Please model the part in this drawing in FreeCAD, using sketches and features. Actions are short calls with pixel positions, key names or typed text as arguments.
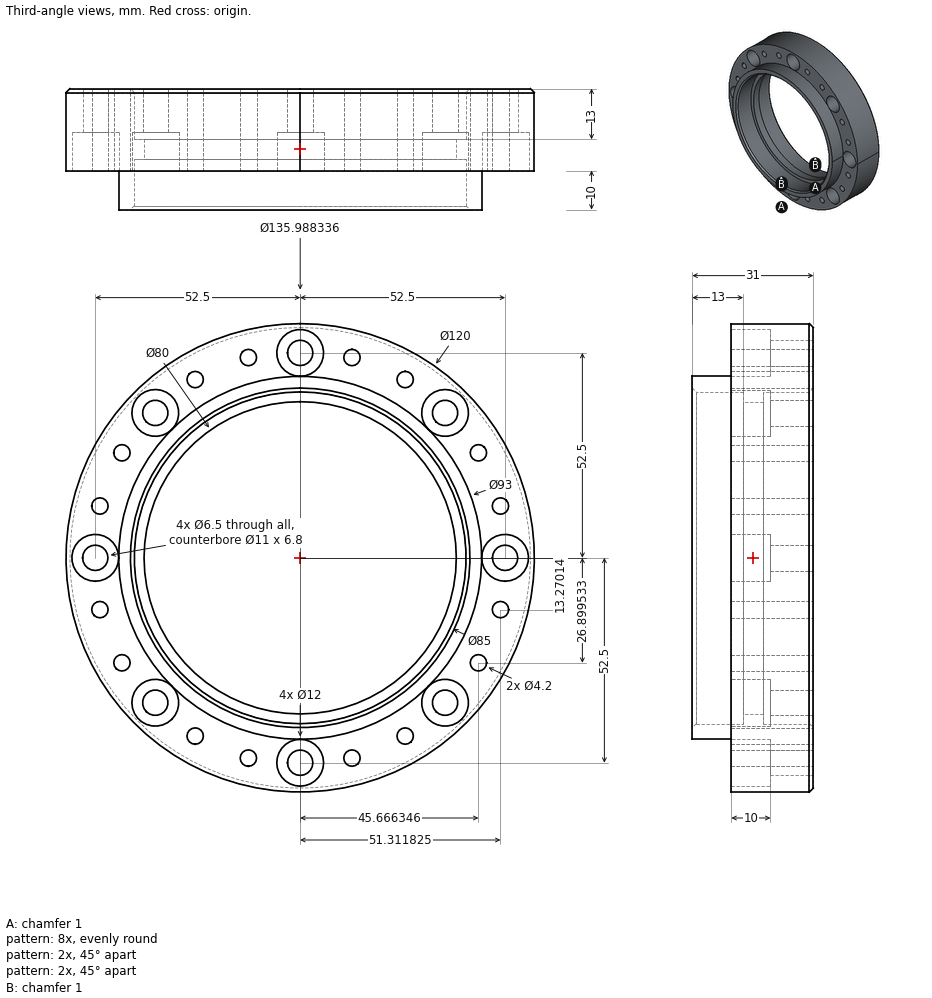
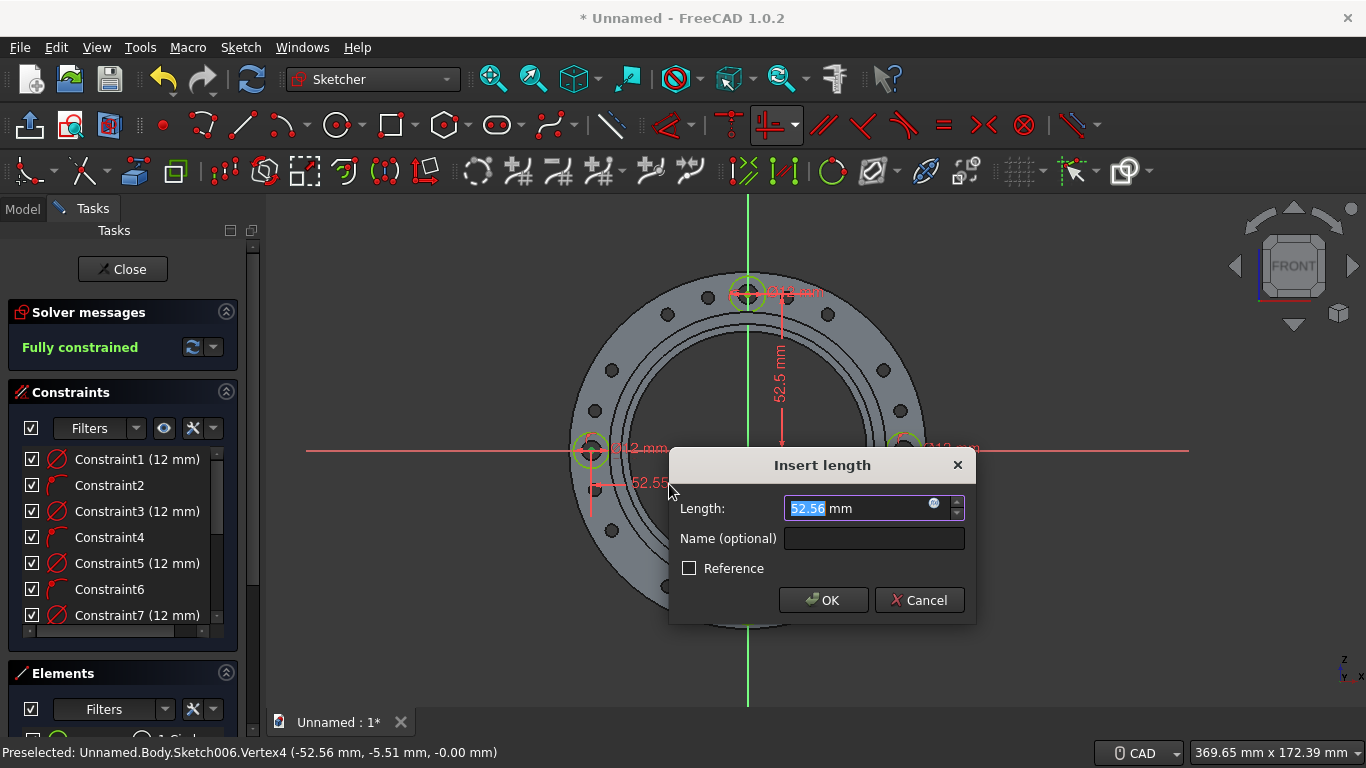
text(52.5)
key(Return)
key(Escape)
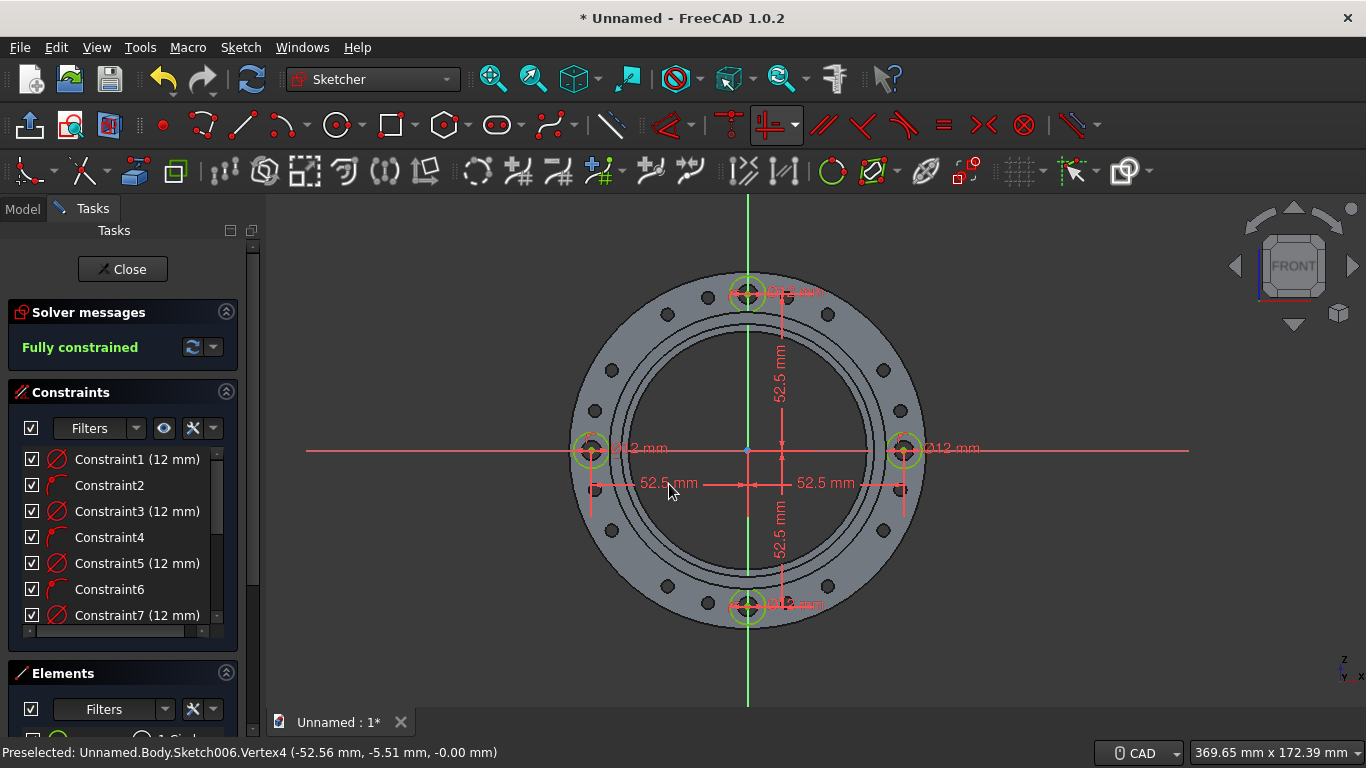
click(123, 269)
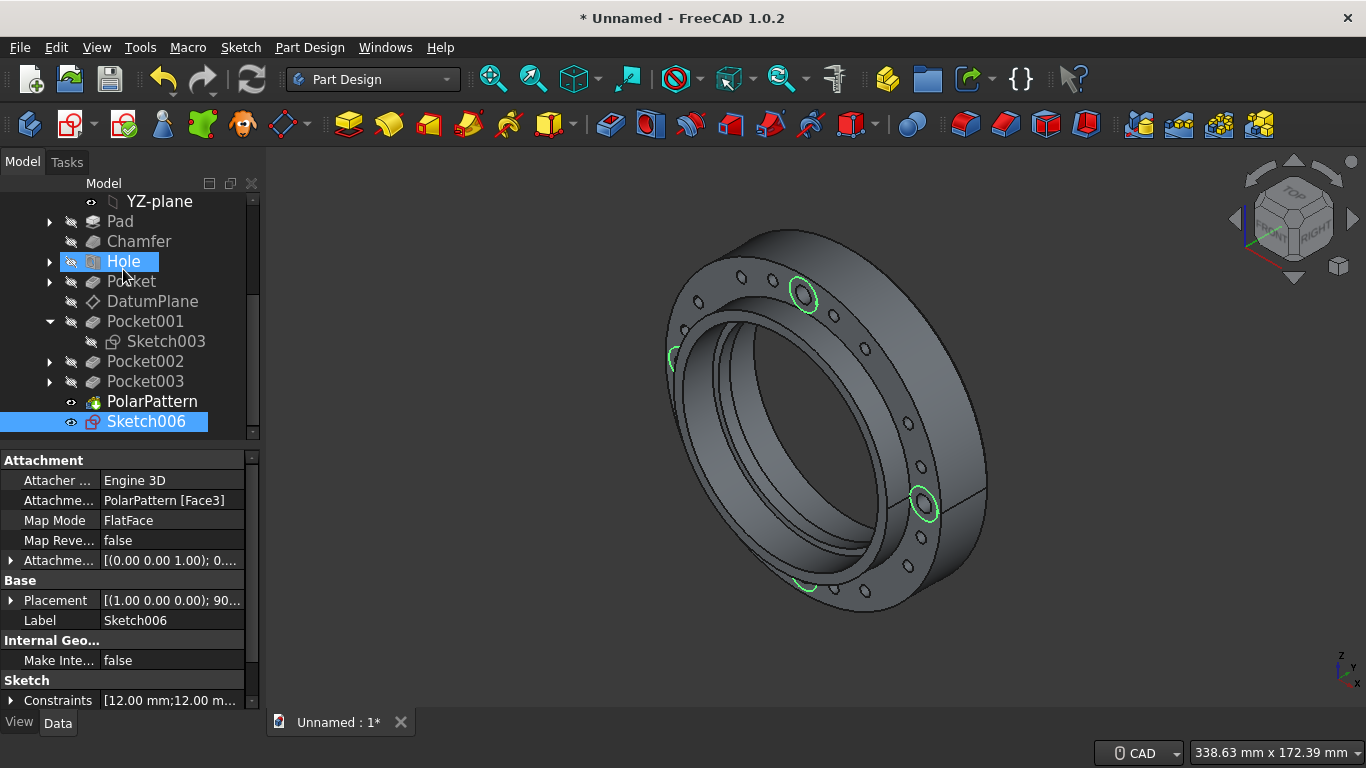
click(612, 124)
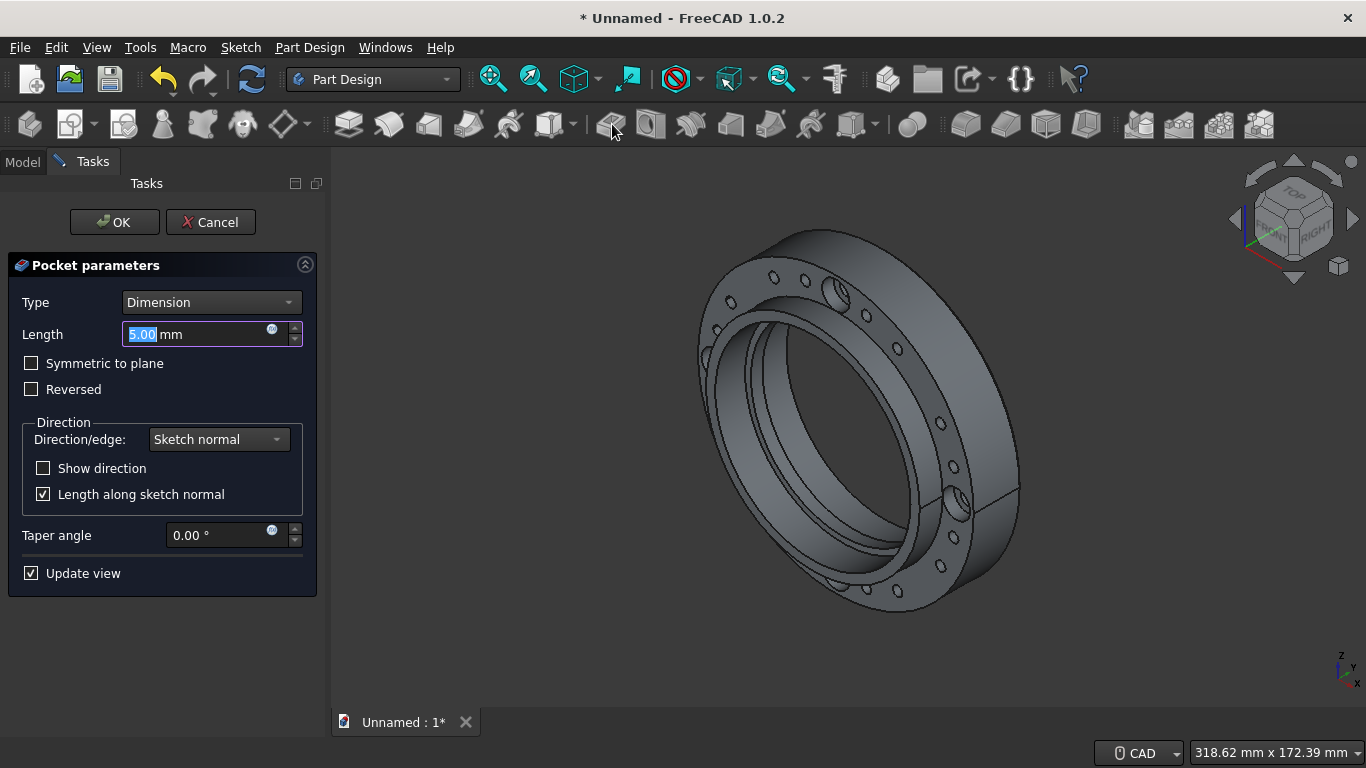
text(10)
key(Tab)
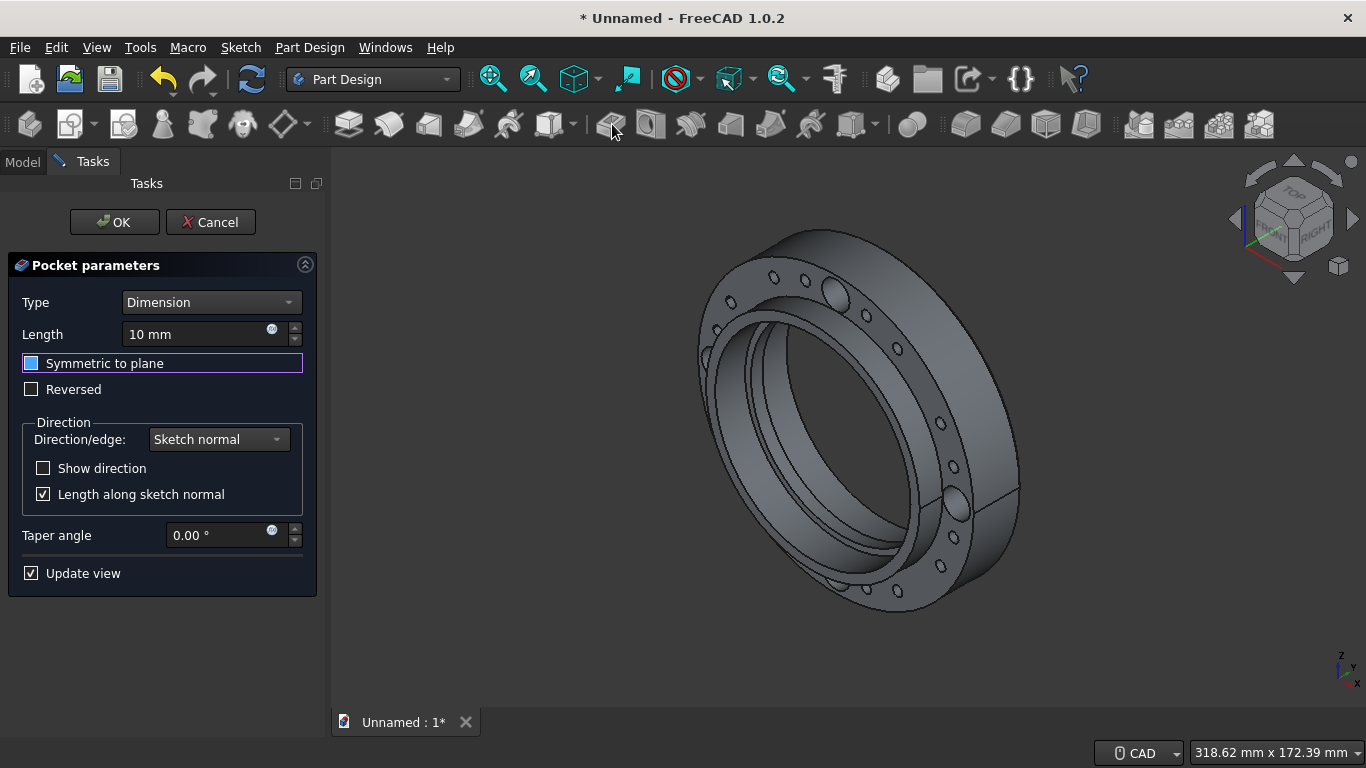
click(115, 222)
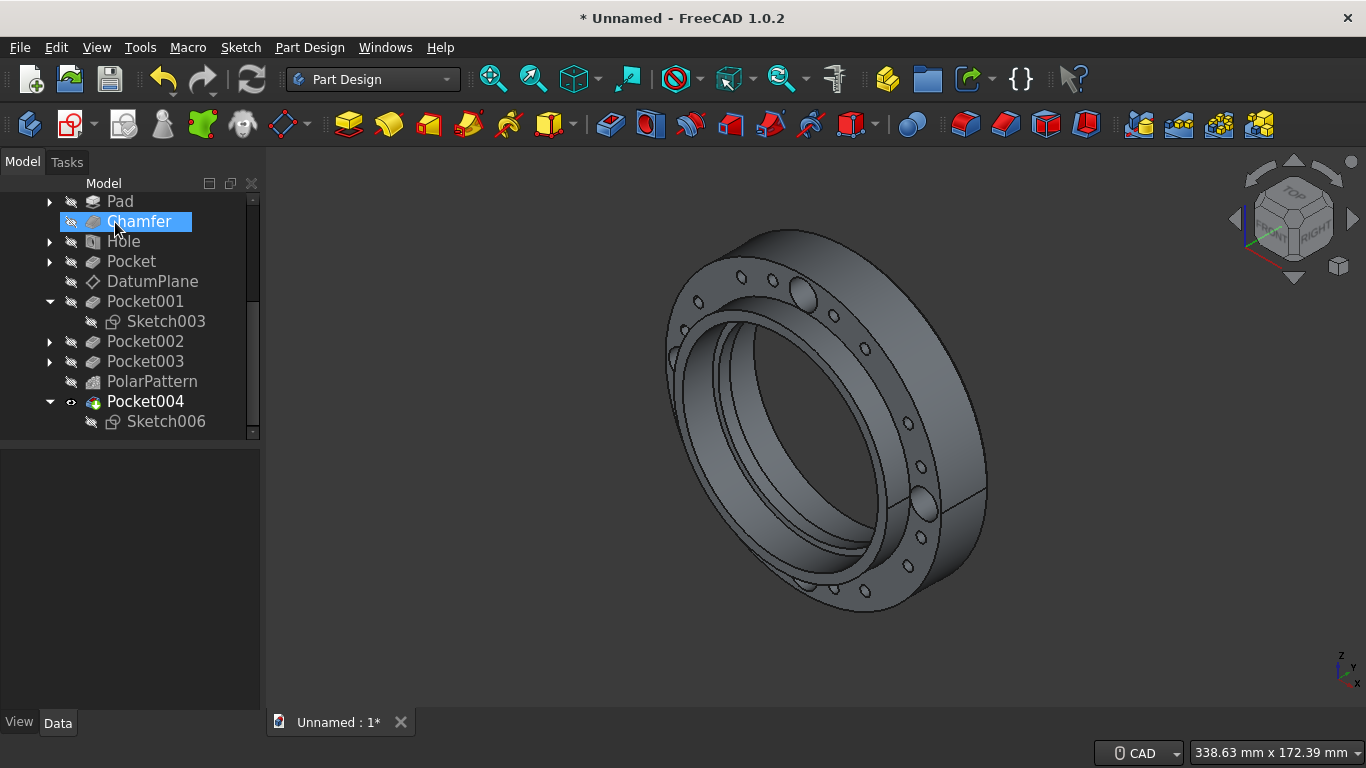
click(116, 242)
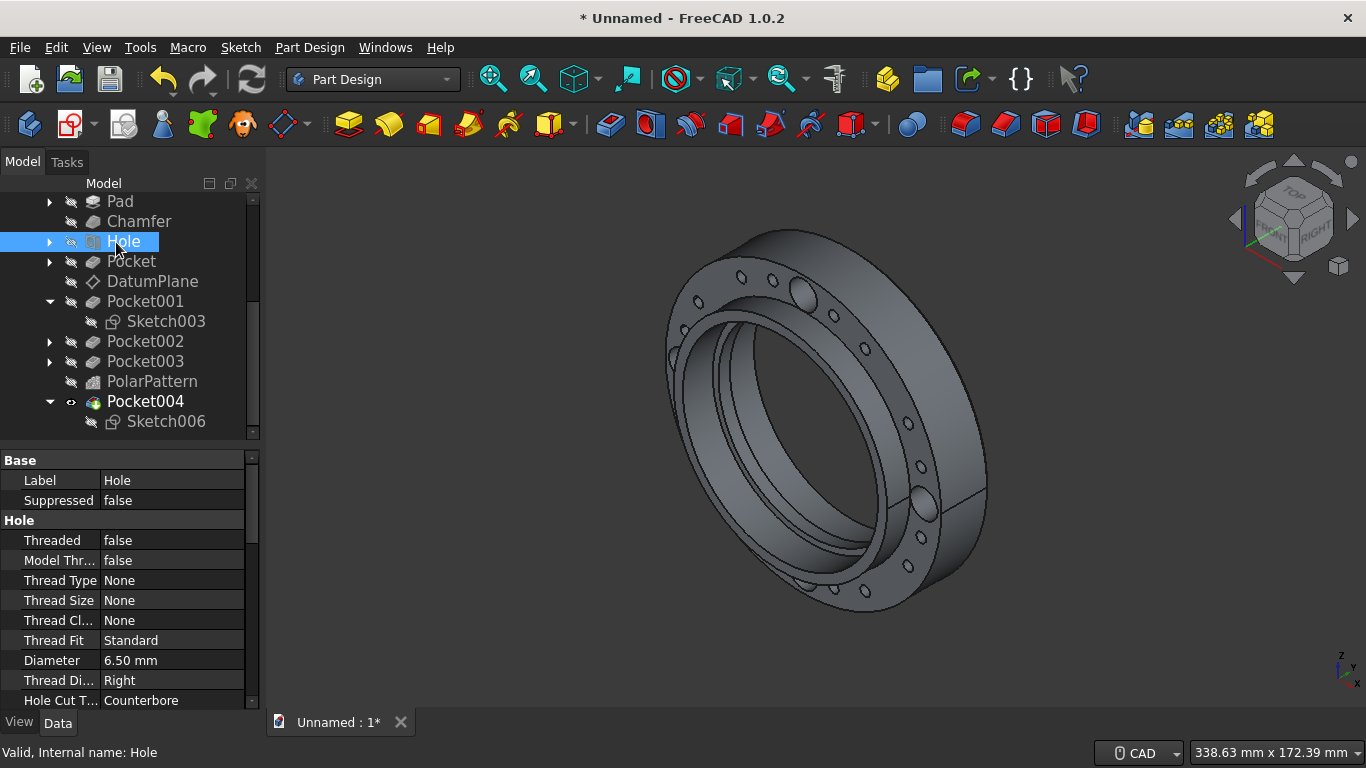
click(1220, 124)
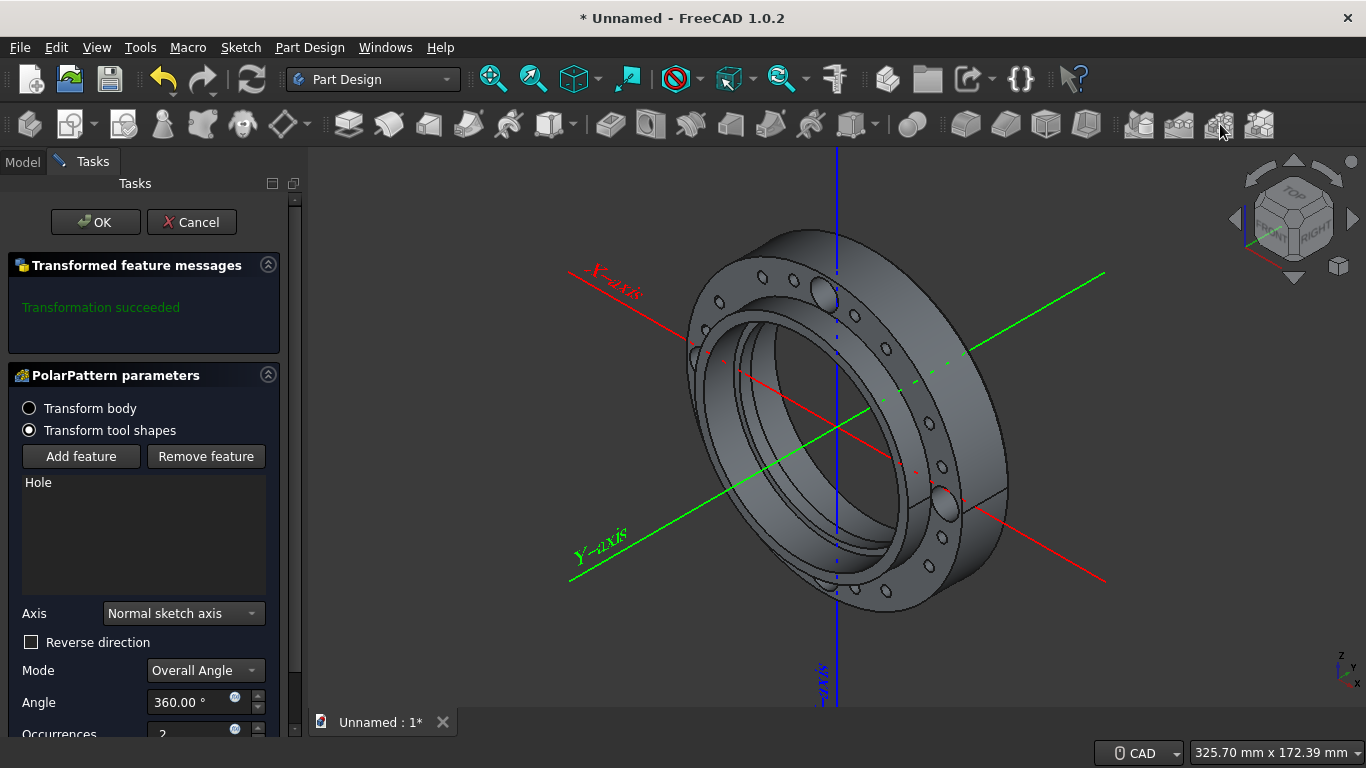
click(184, 614)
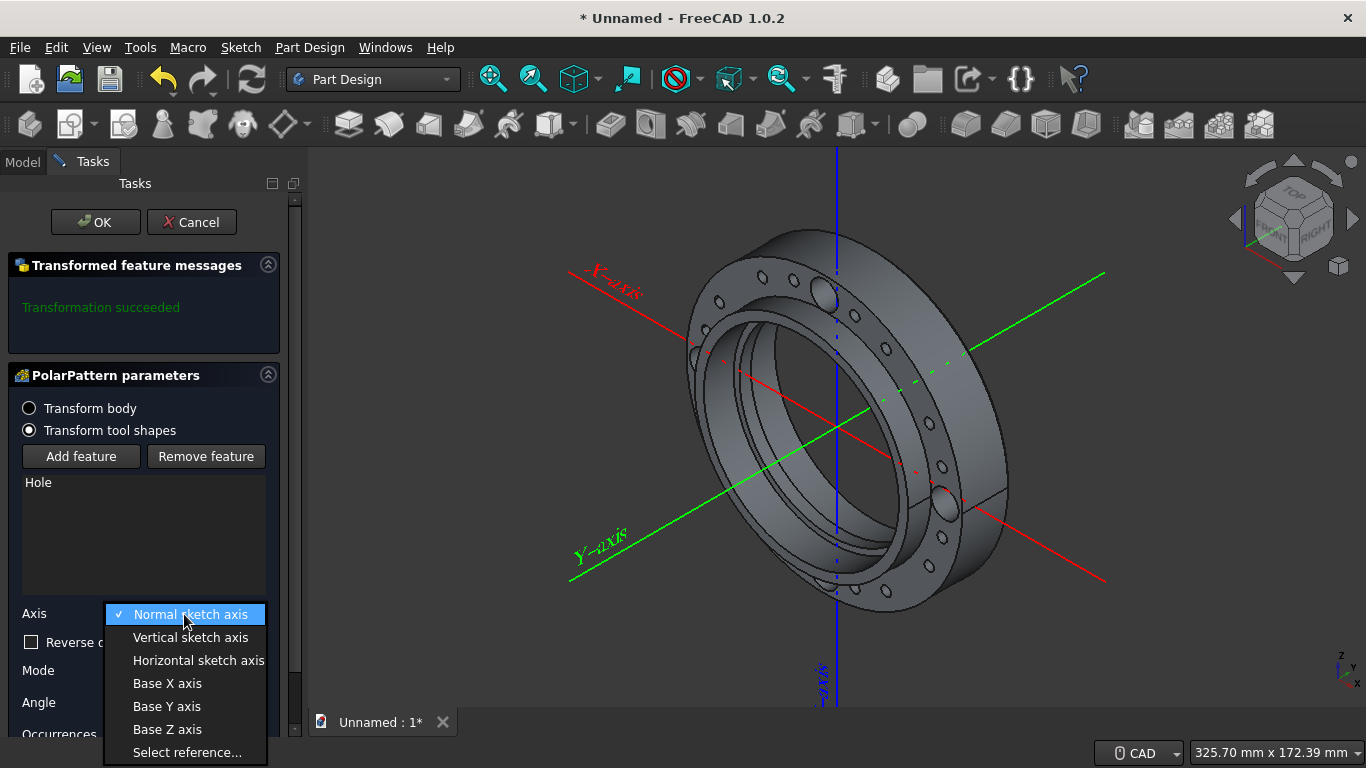
click(184, 706)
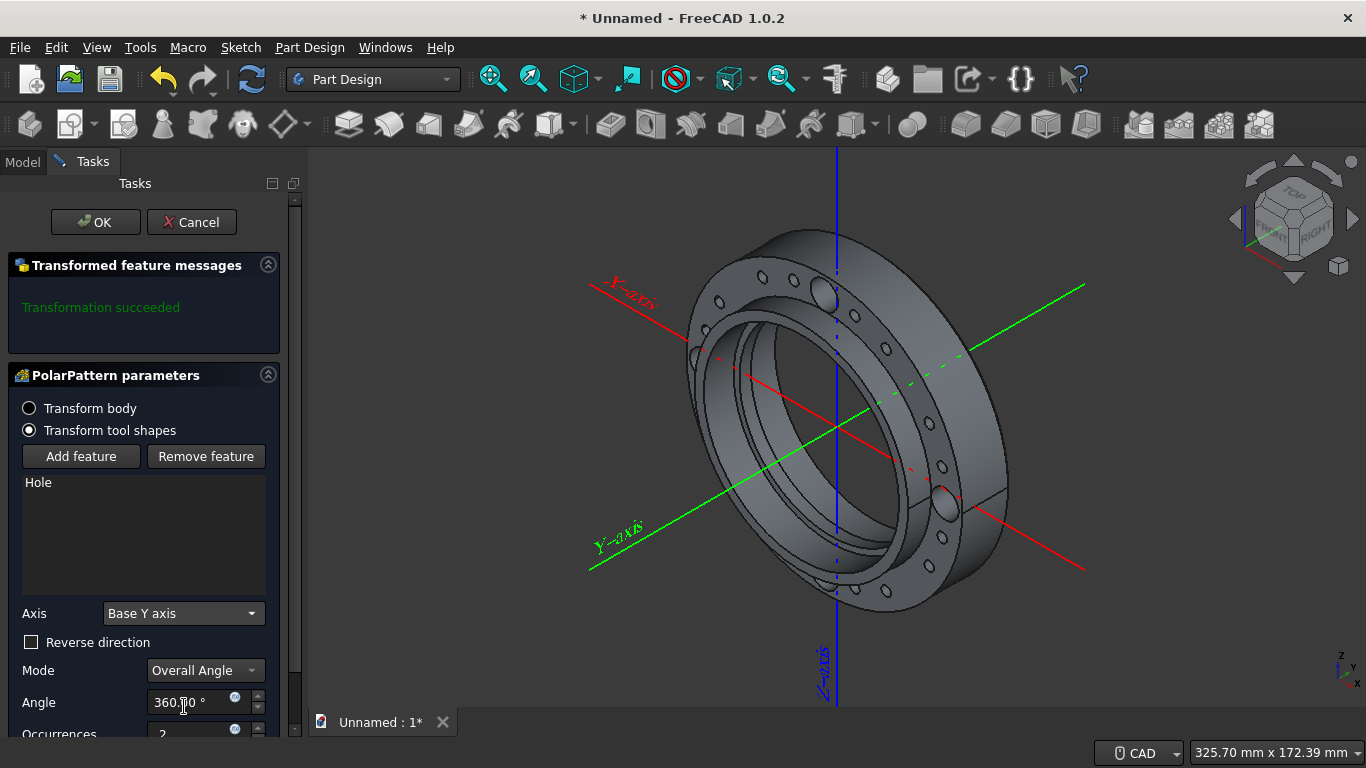
click(206, 670)